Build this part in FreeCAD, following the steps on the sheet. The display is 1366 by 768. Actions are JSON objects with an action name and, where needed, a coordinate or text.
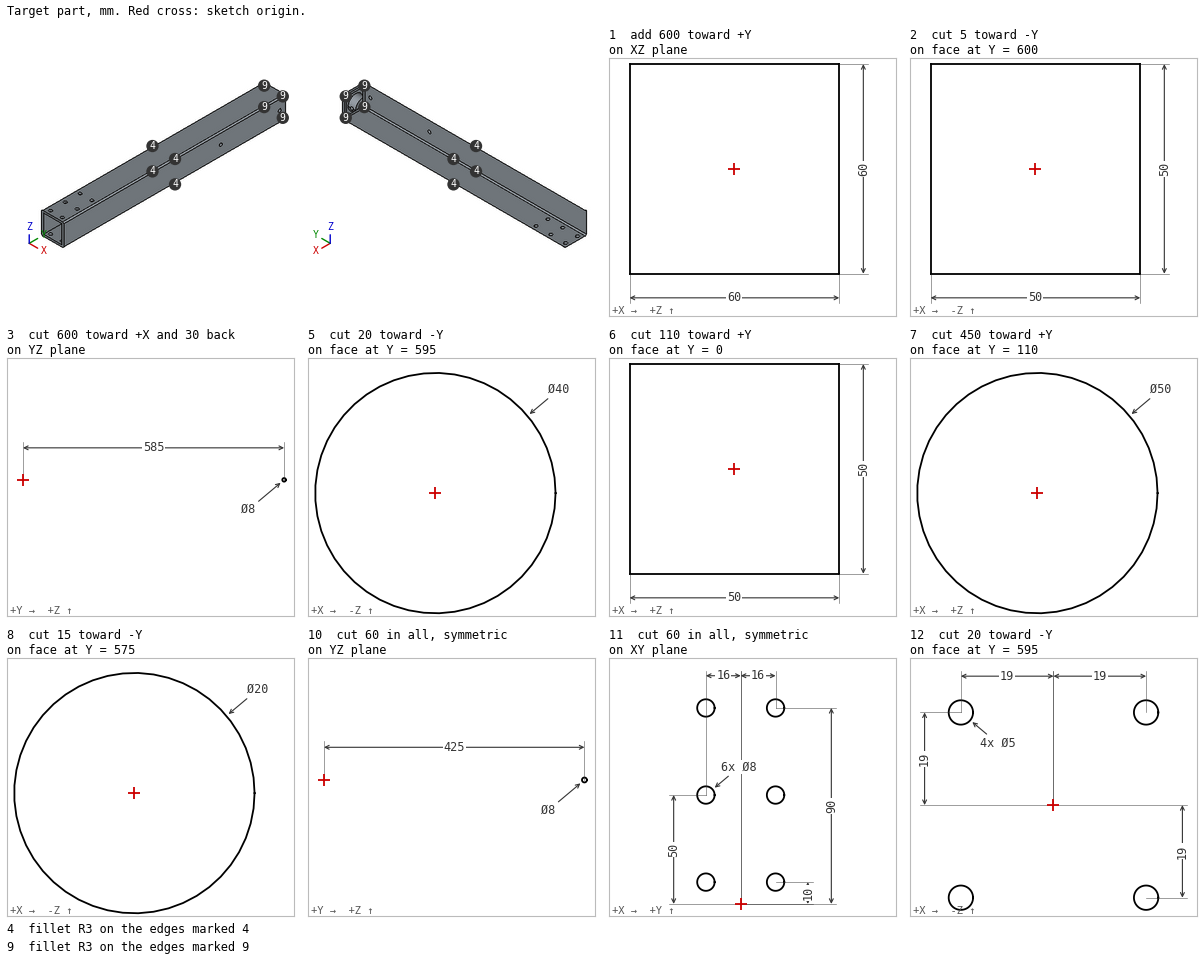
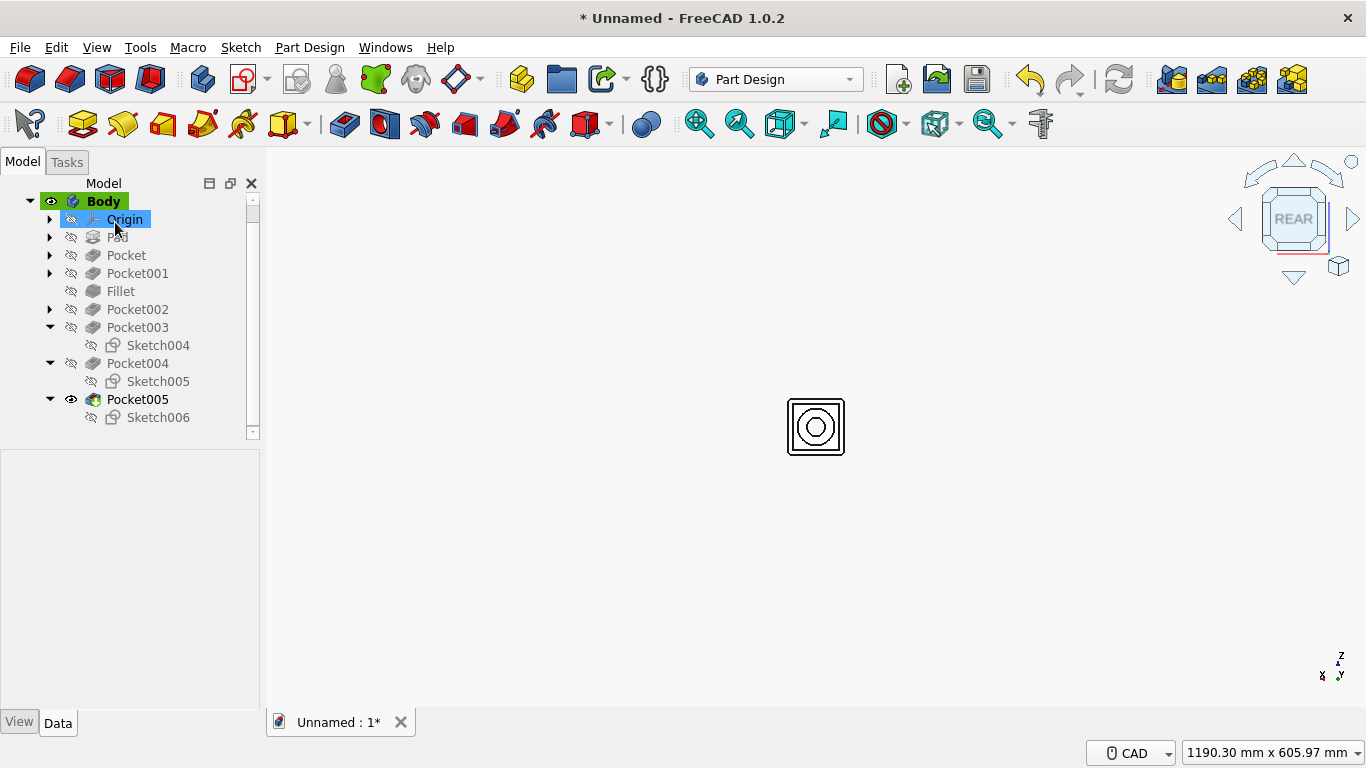
{"action": "scroll", "coordinate": [793, 449], "scroll_direction": "up", "scroll_amount": 11}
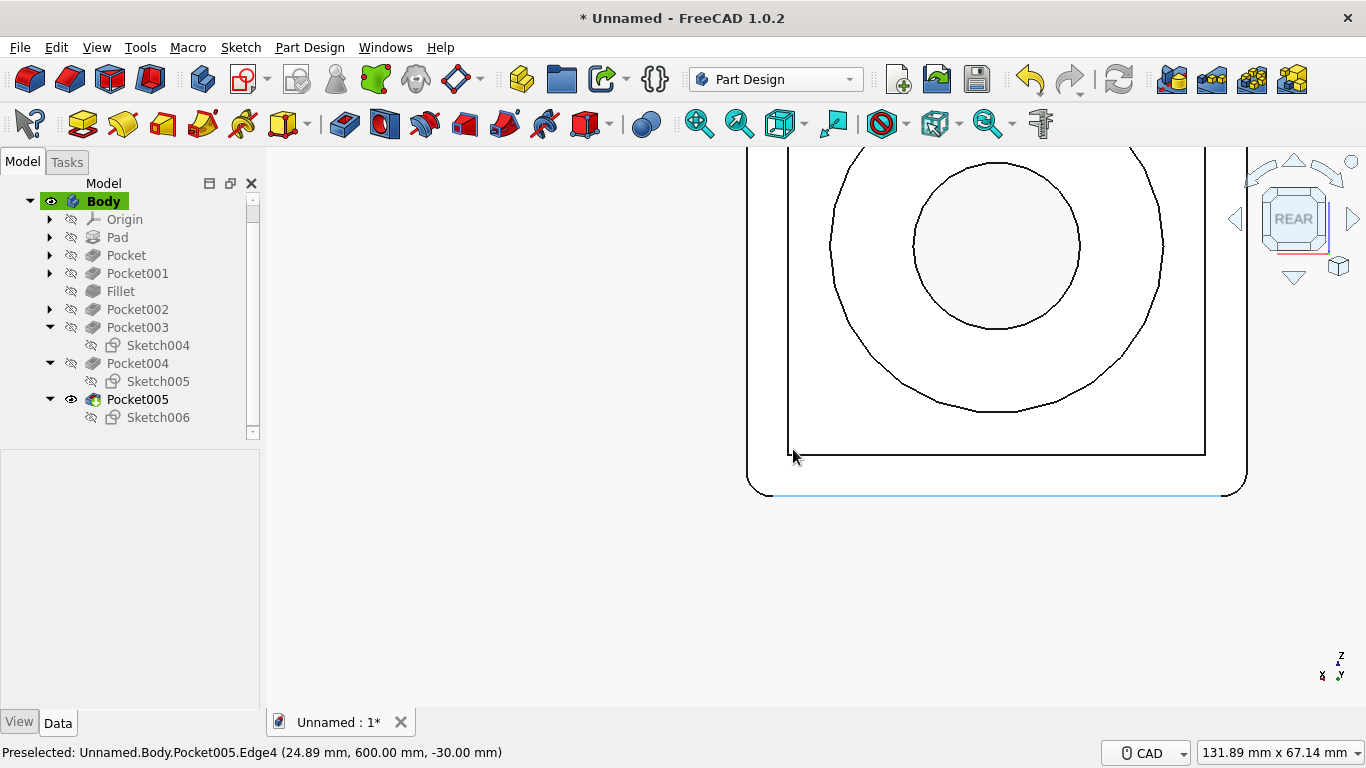
{"action": "key", "text": "v f"}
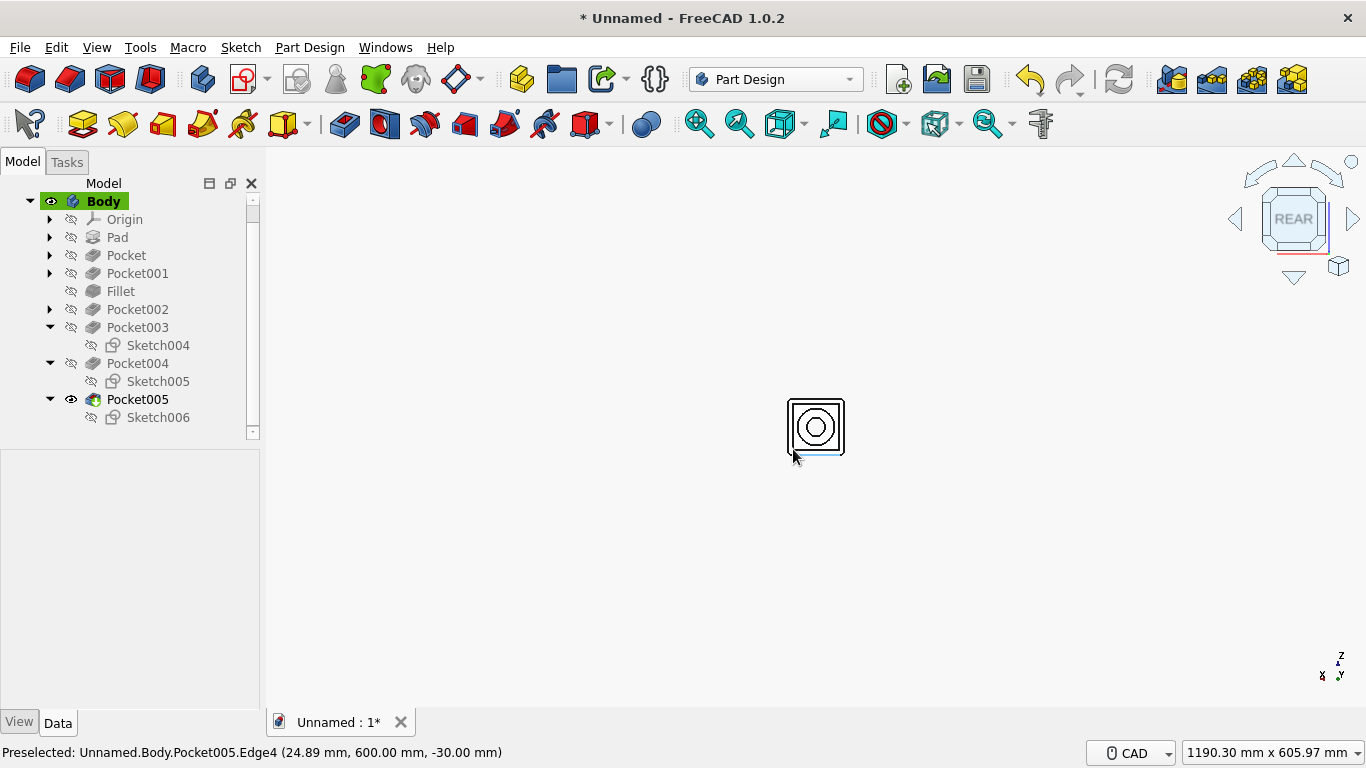
{"action": "key", "text": "0"}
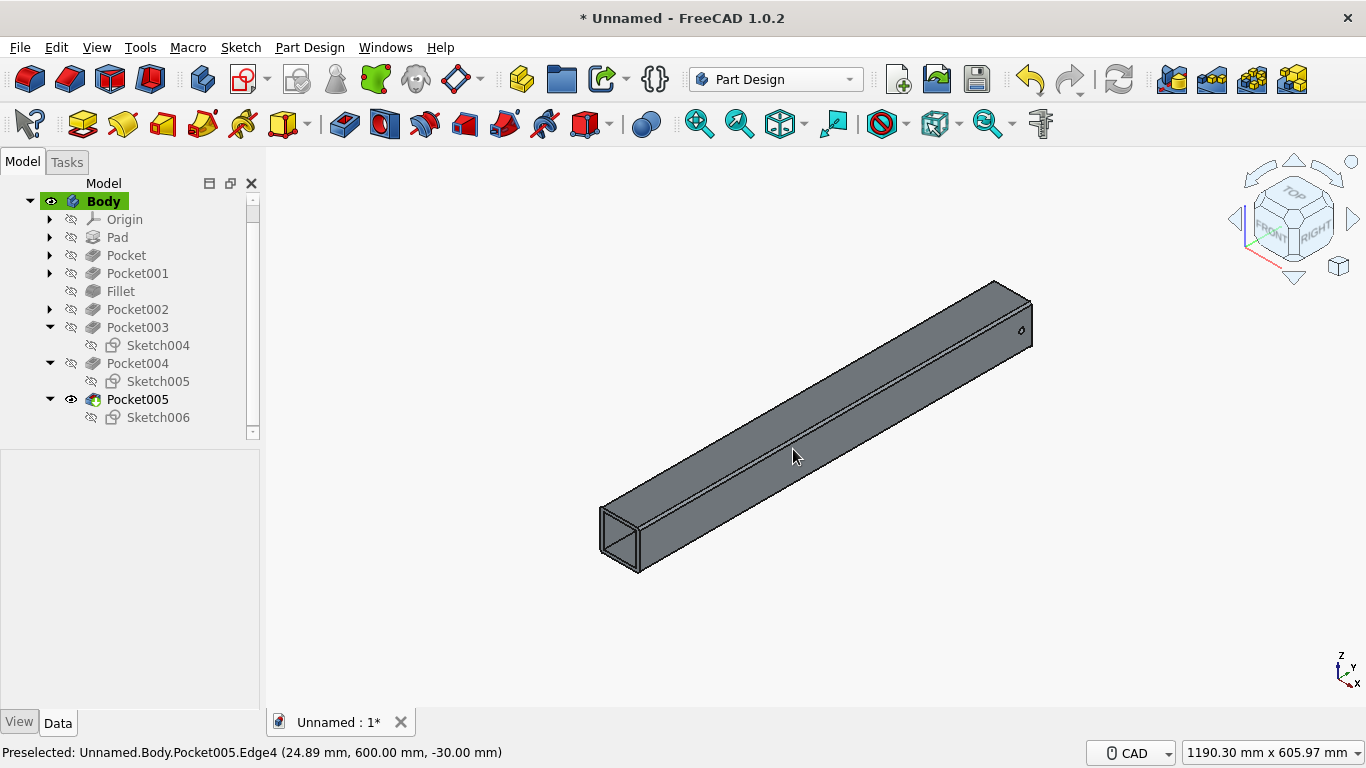
{"action": "scroll", "coordinate": [1027, 342], "scroll_direction": "up", "scroll_amount": 11}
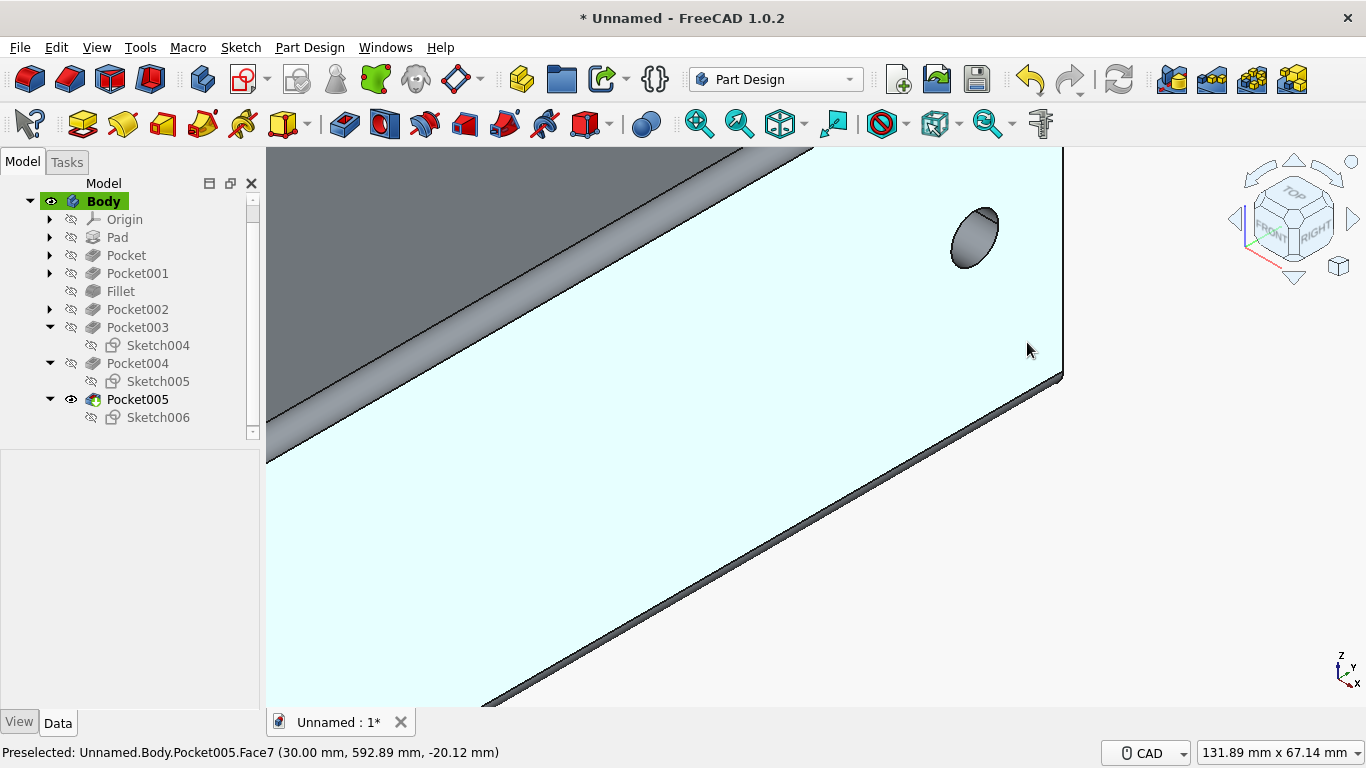
{"action": "left_click", "coordinate": [700, 124]}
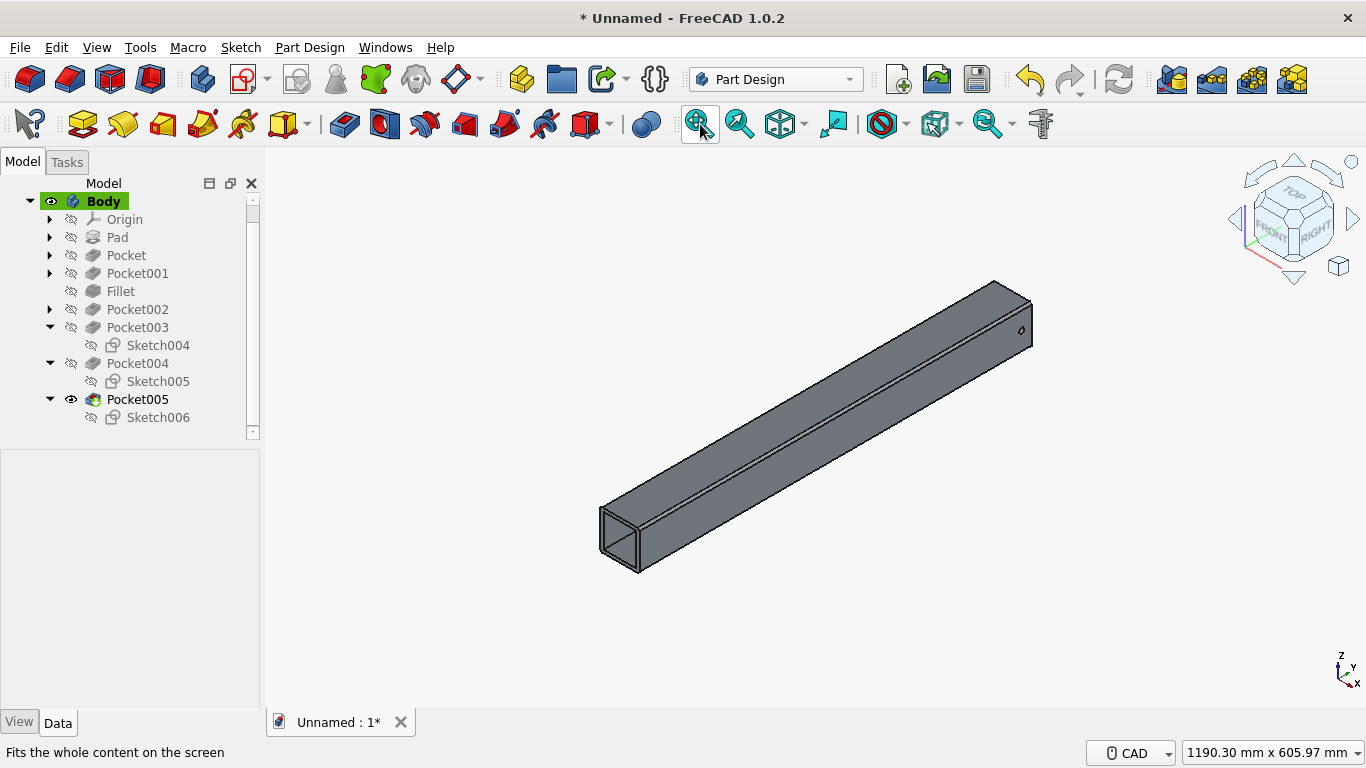
{"action": "key", "text": "2"}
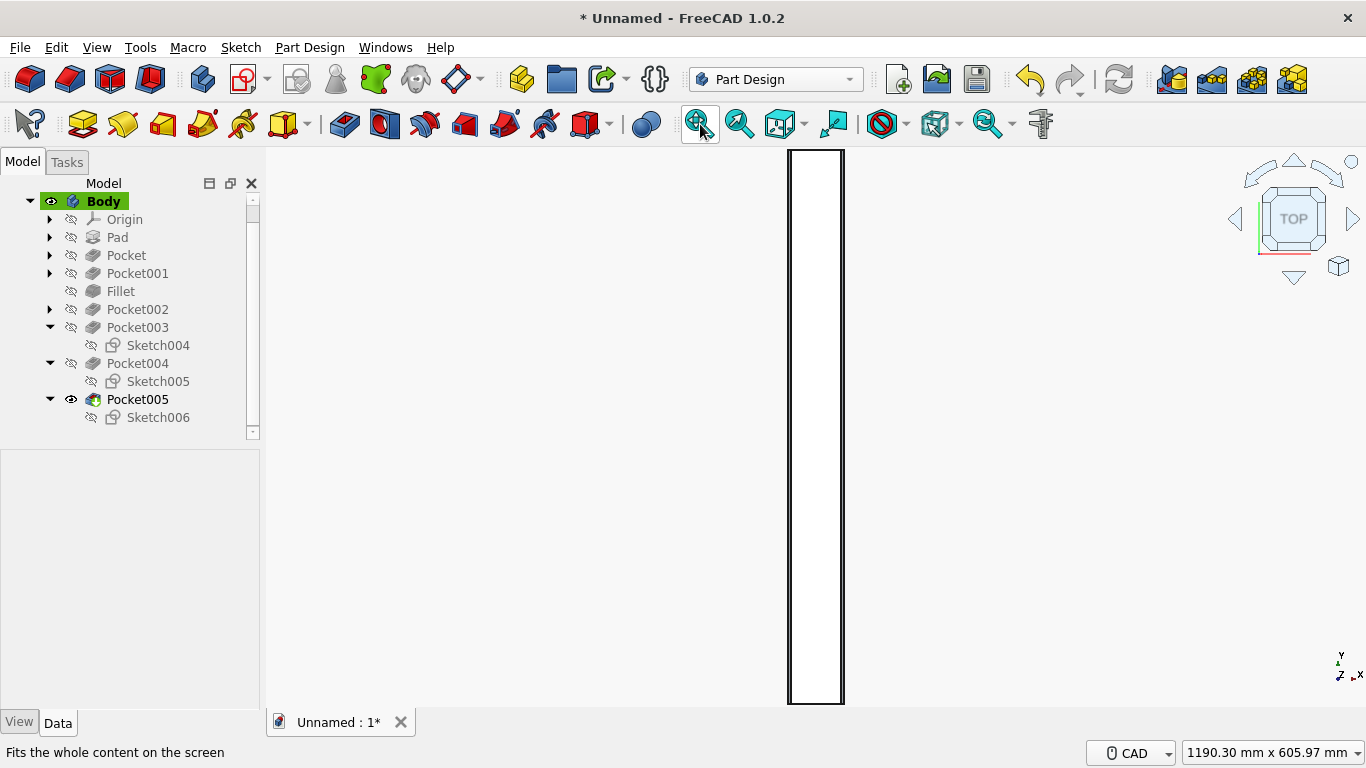
{"action": "key", "text": "1"}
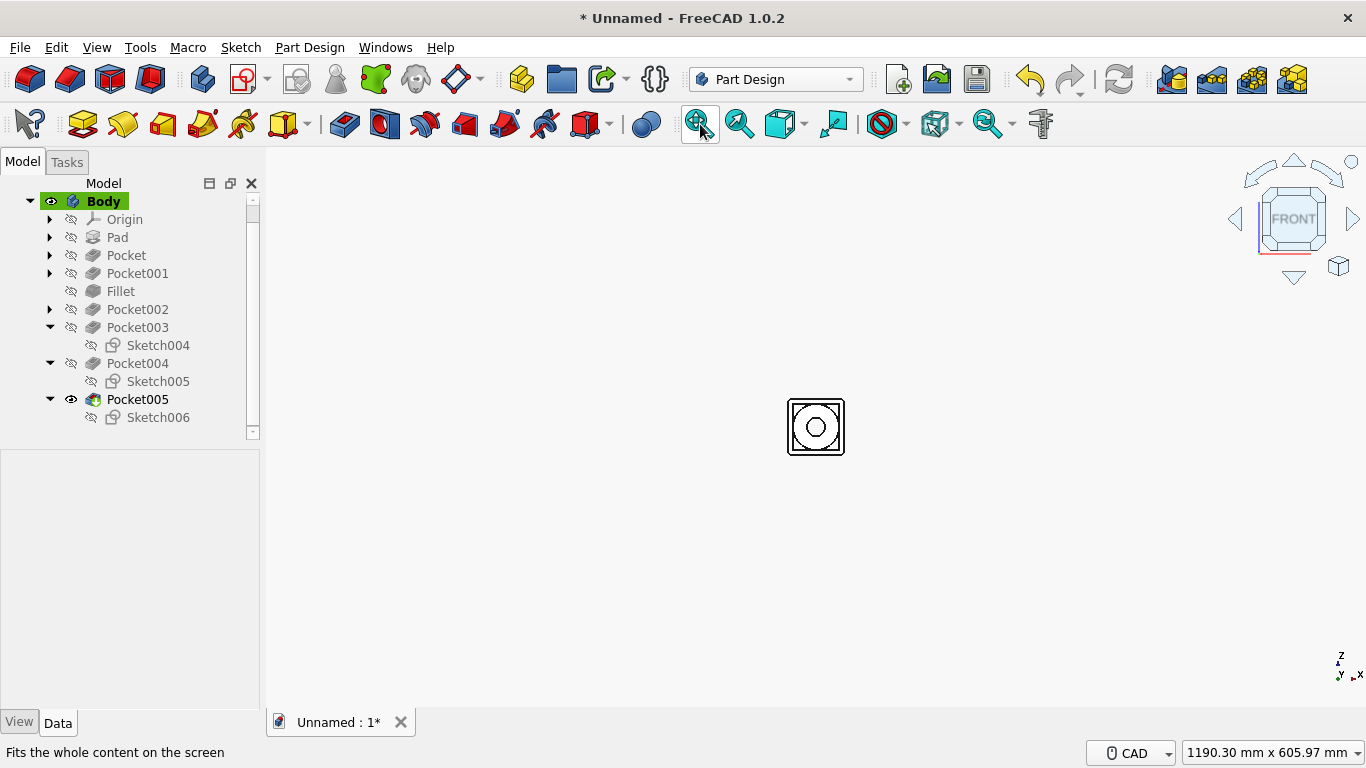
{"action": "left_click", "coordinate": [700, 124]}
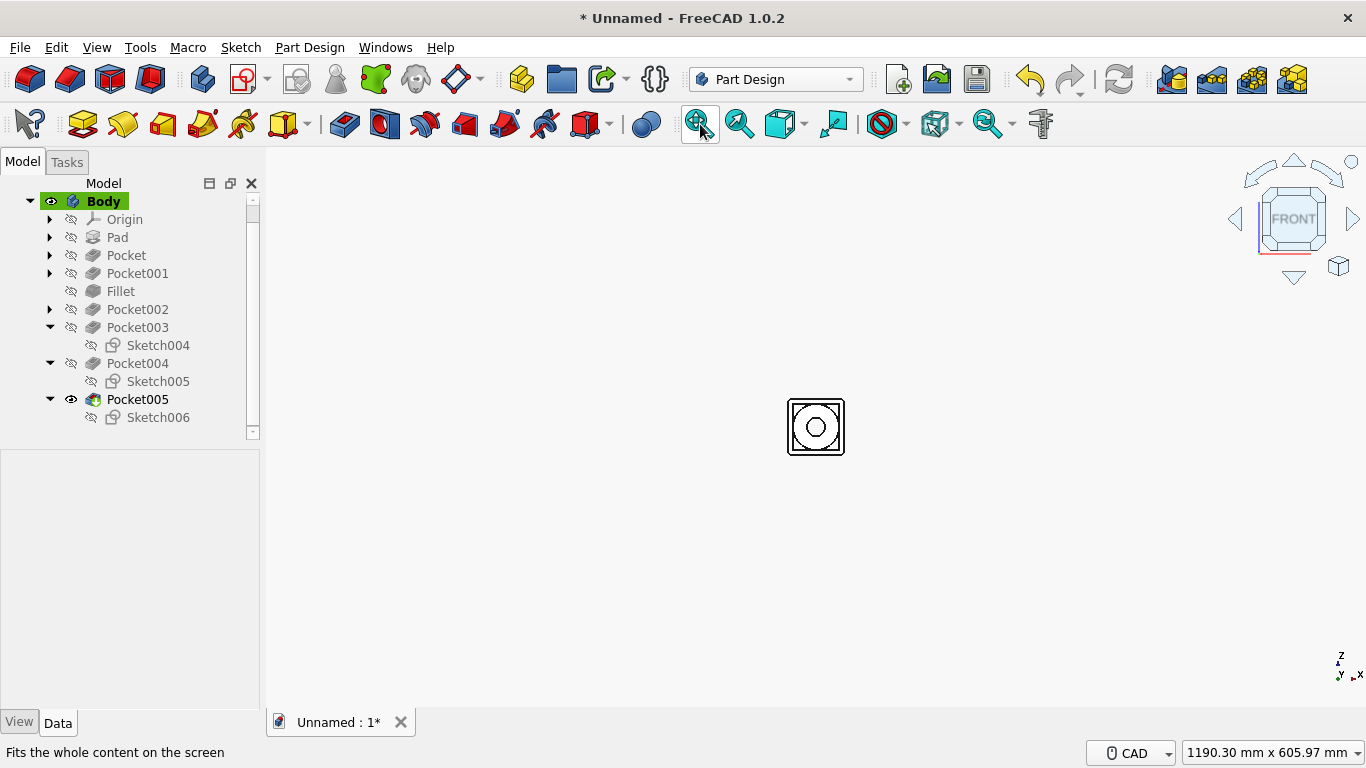
{"action": "scroll", "coordinate": [839, 449], "scroll_direction": "up", "scroll_amount": 11}